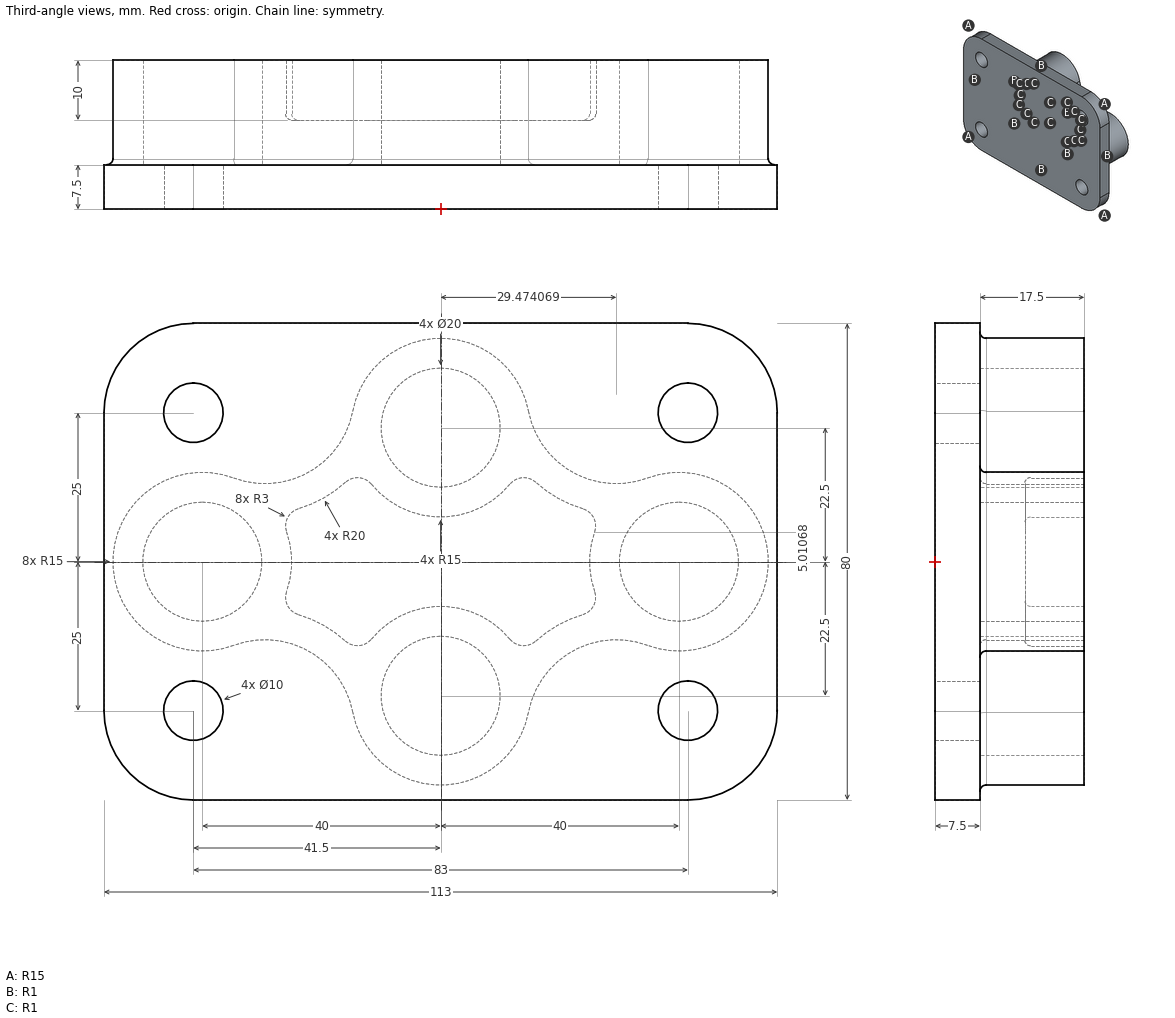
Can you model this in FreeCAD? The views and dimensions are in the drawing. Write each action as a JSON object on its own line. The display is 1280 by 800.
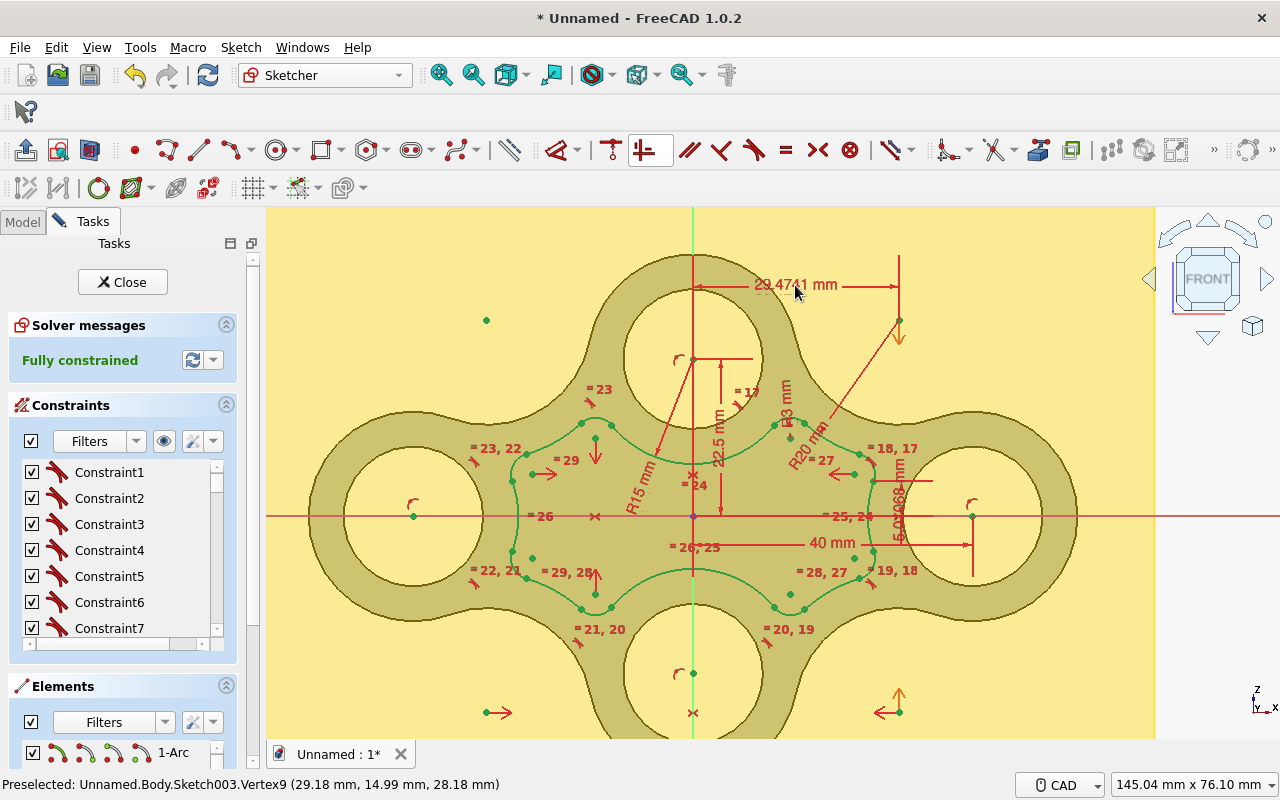
{"action": "left_click", "coordinate": [123, 282]}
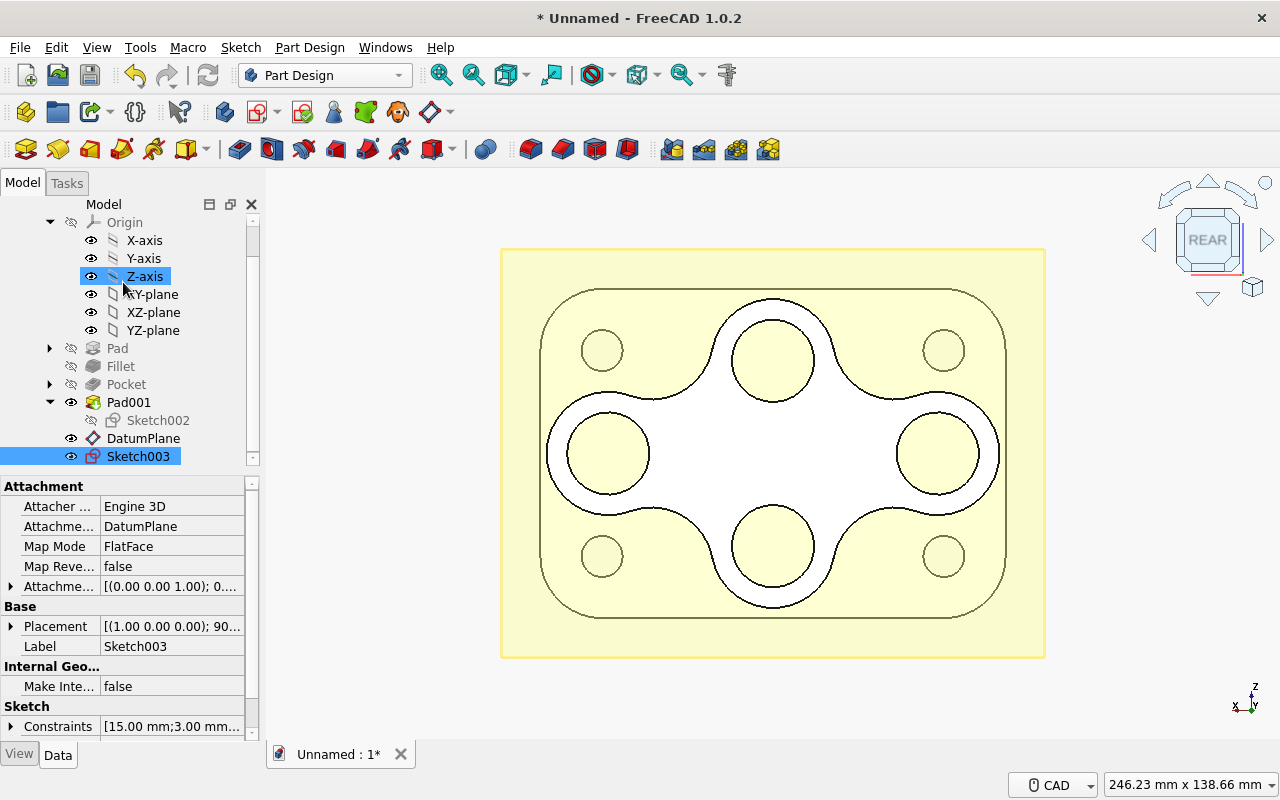
{"action": "left_click", "coordinate": [240, 150]}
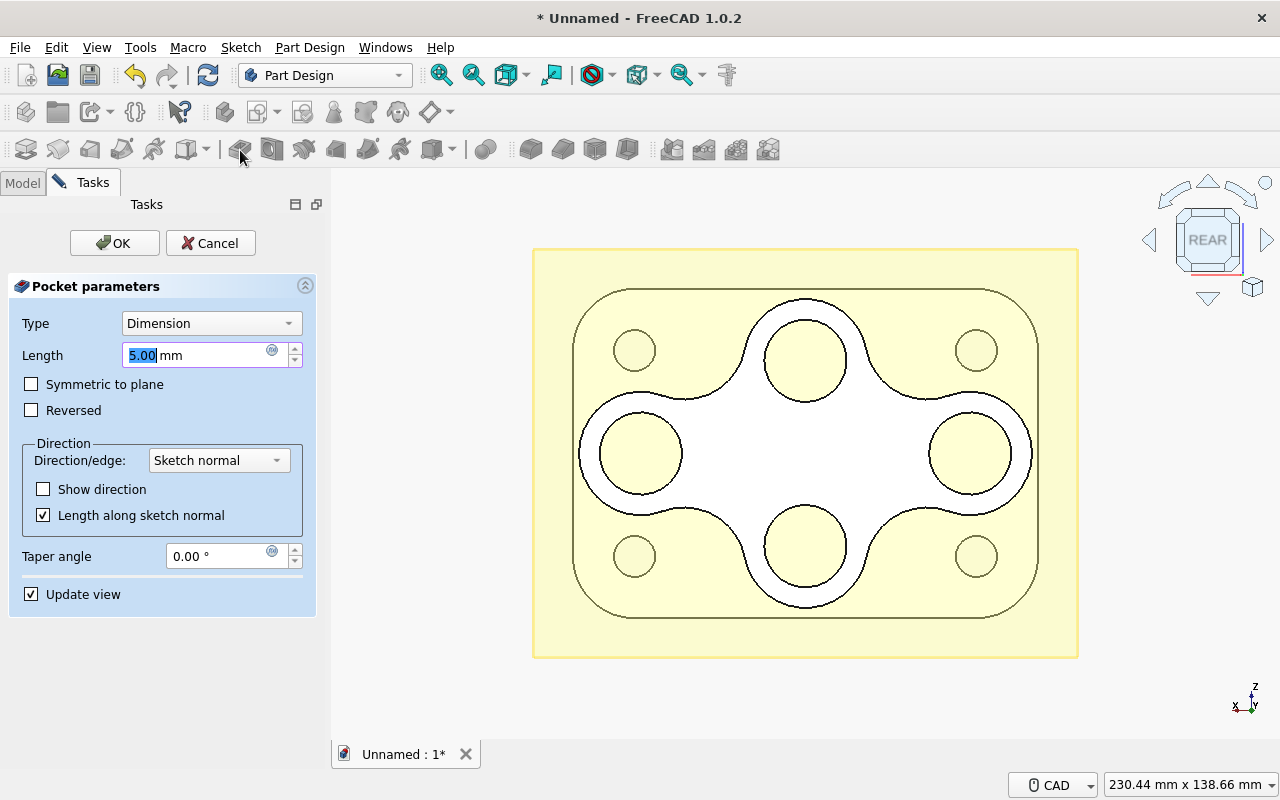
{"action": "type", "text": "10"}
{"action": "key", "text": "Tab"}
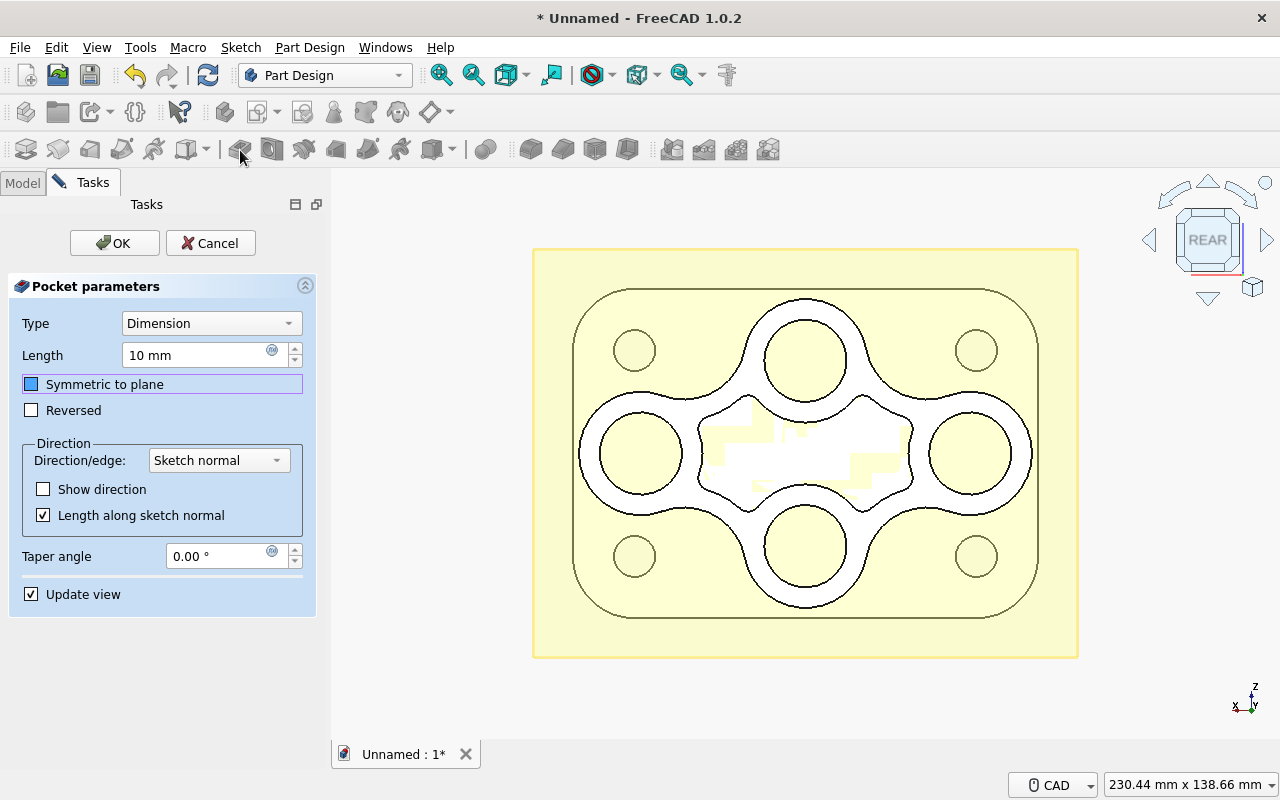
{"action": "left_click", "coordinate": [115, 243]}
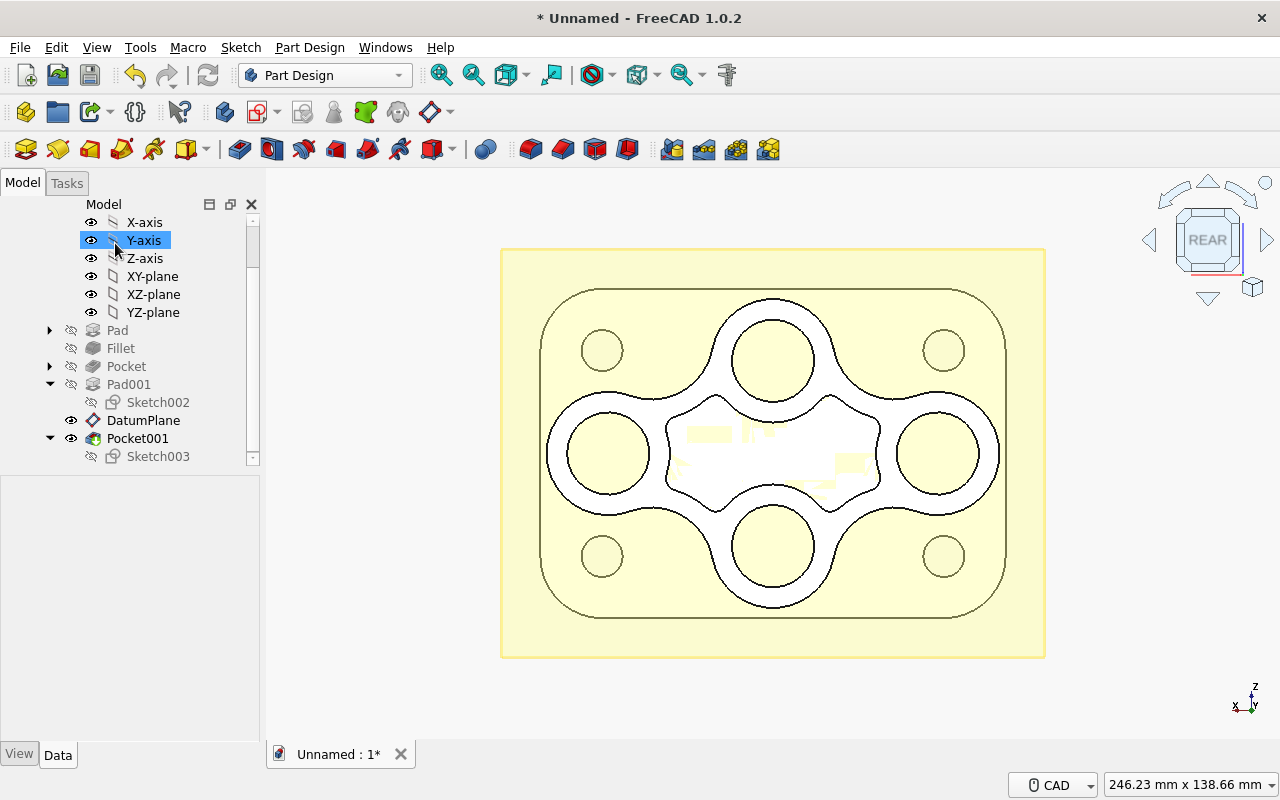
{"action": "left_click", "coordinate": [116, 420]}
{"action": "key", "text": "space"}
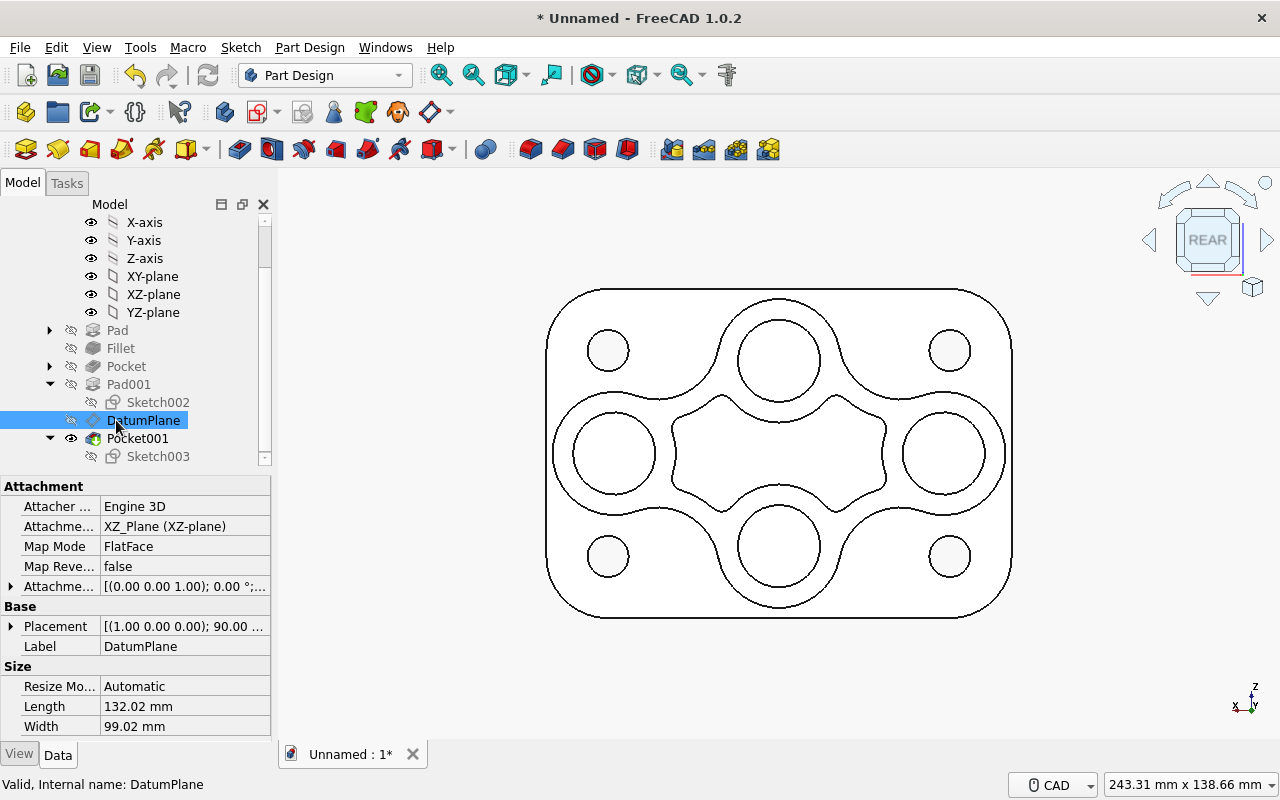
{"action": "key", "text": "0"}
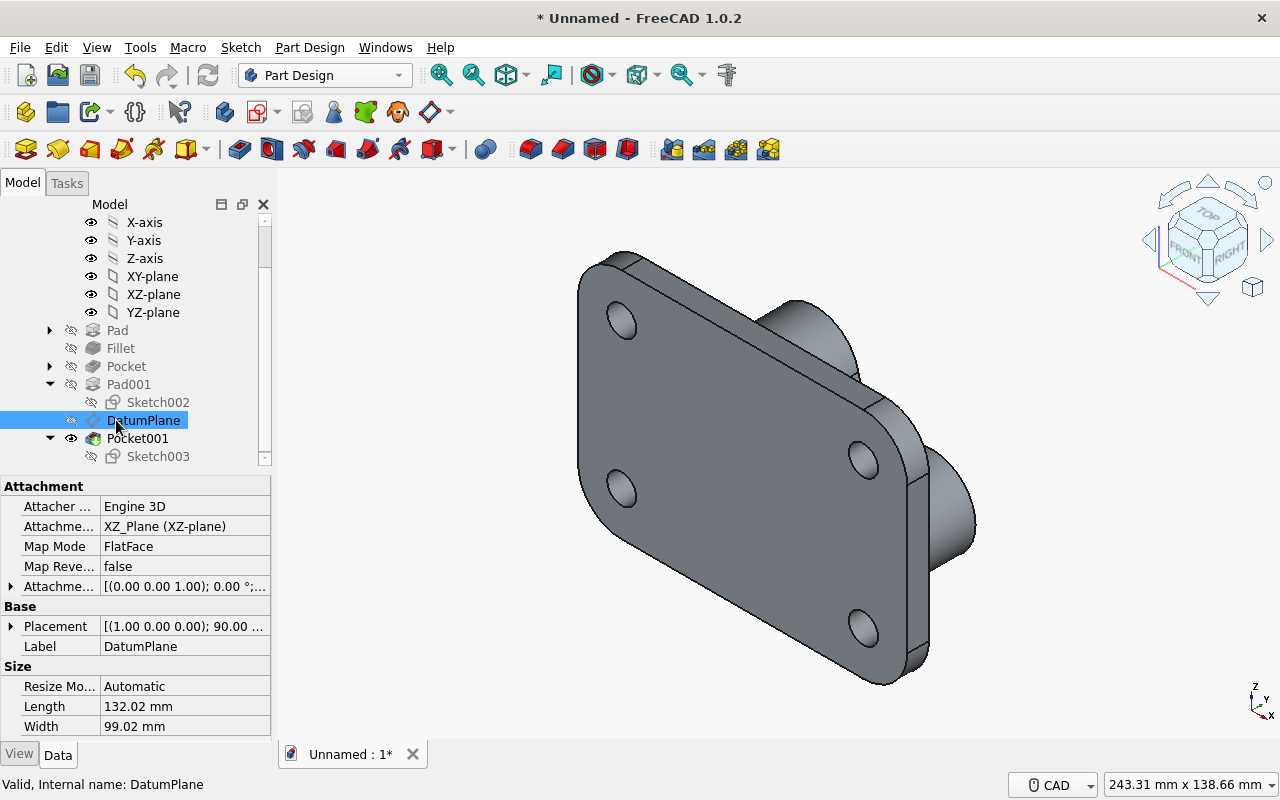
{"action": "key", "text": "2"}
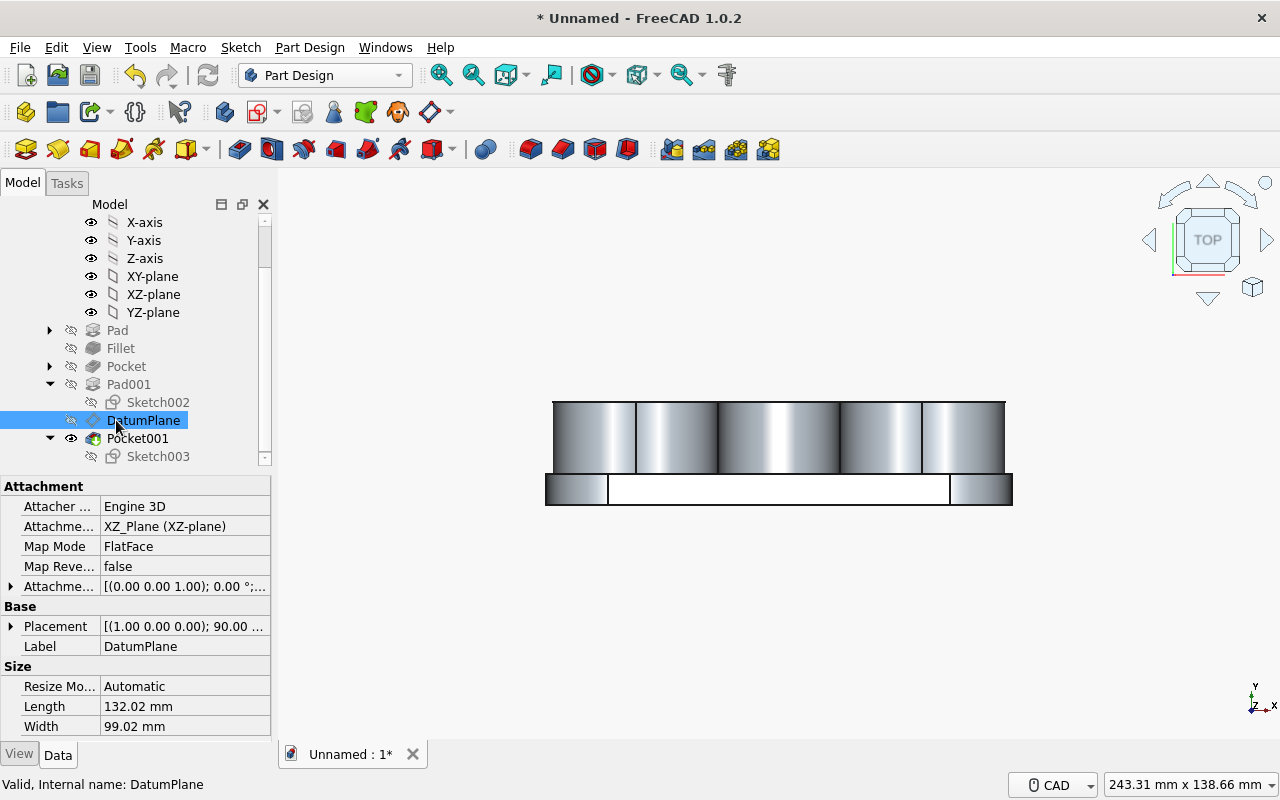
{"action": "key", "text": "1"}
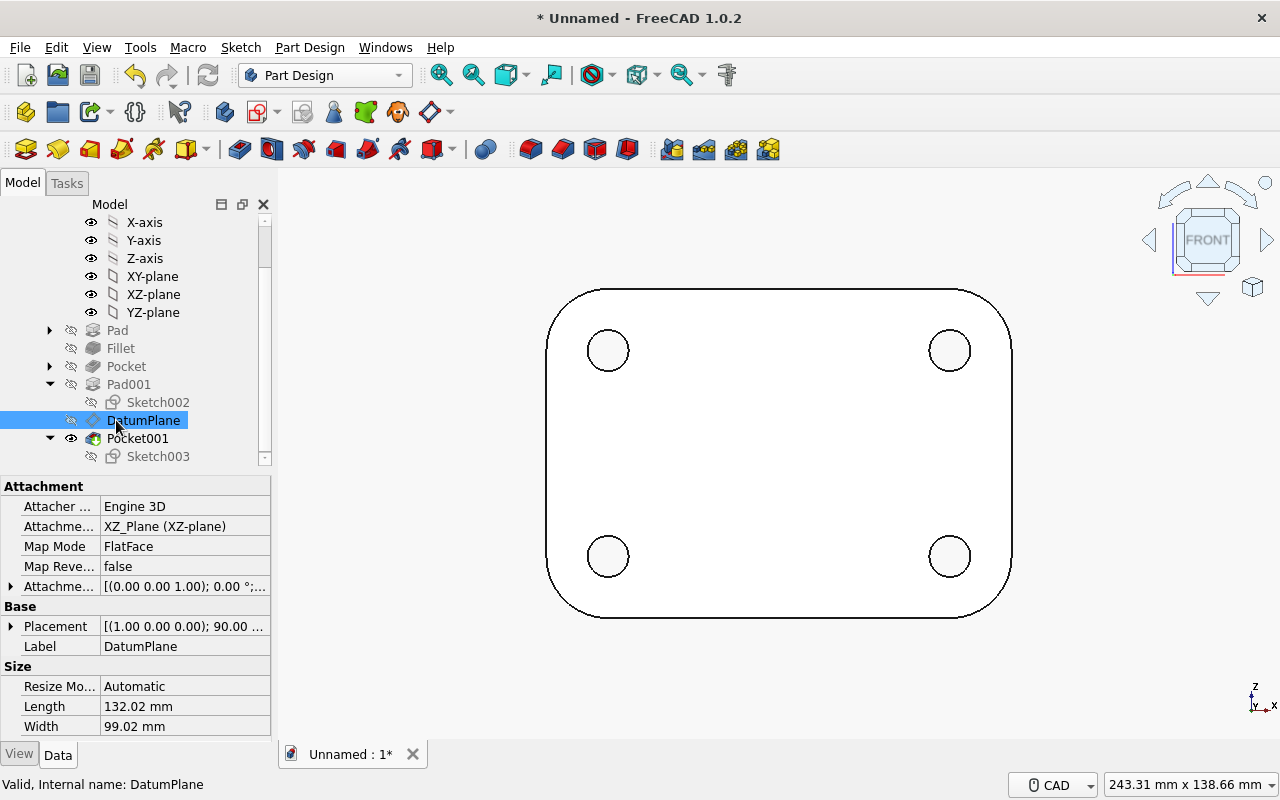
{"action": "key", "text": "3"}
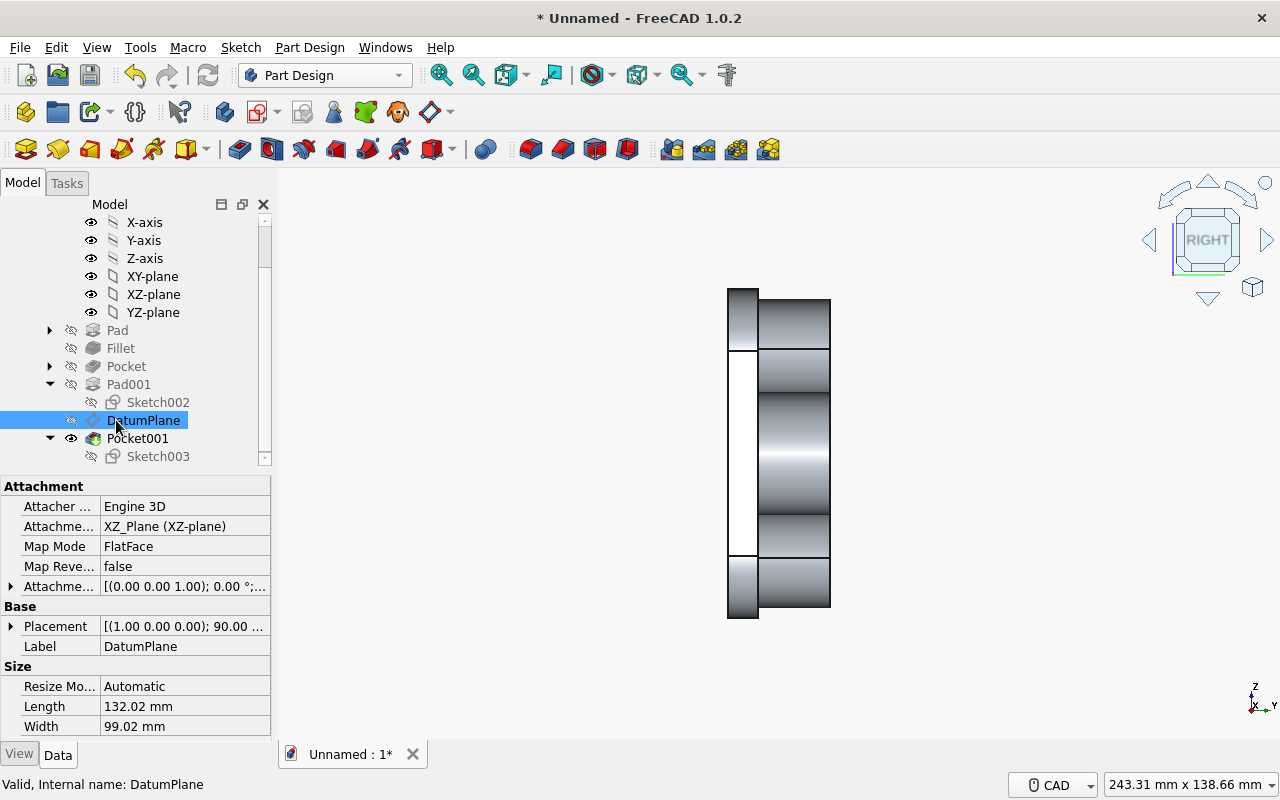
{"action": "key", "text": "5"}